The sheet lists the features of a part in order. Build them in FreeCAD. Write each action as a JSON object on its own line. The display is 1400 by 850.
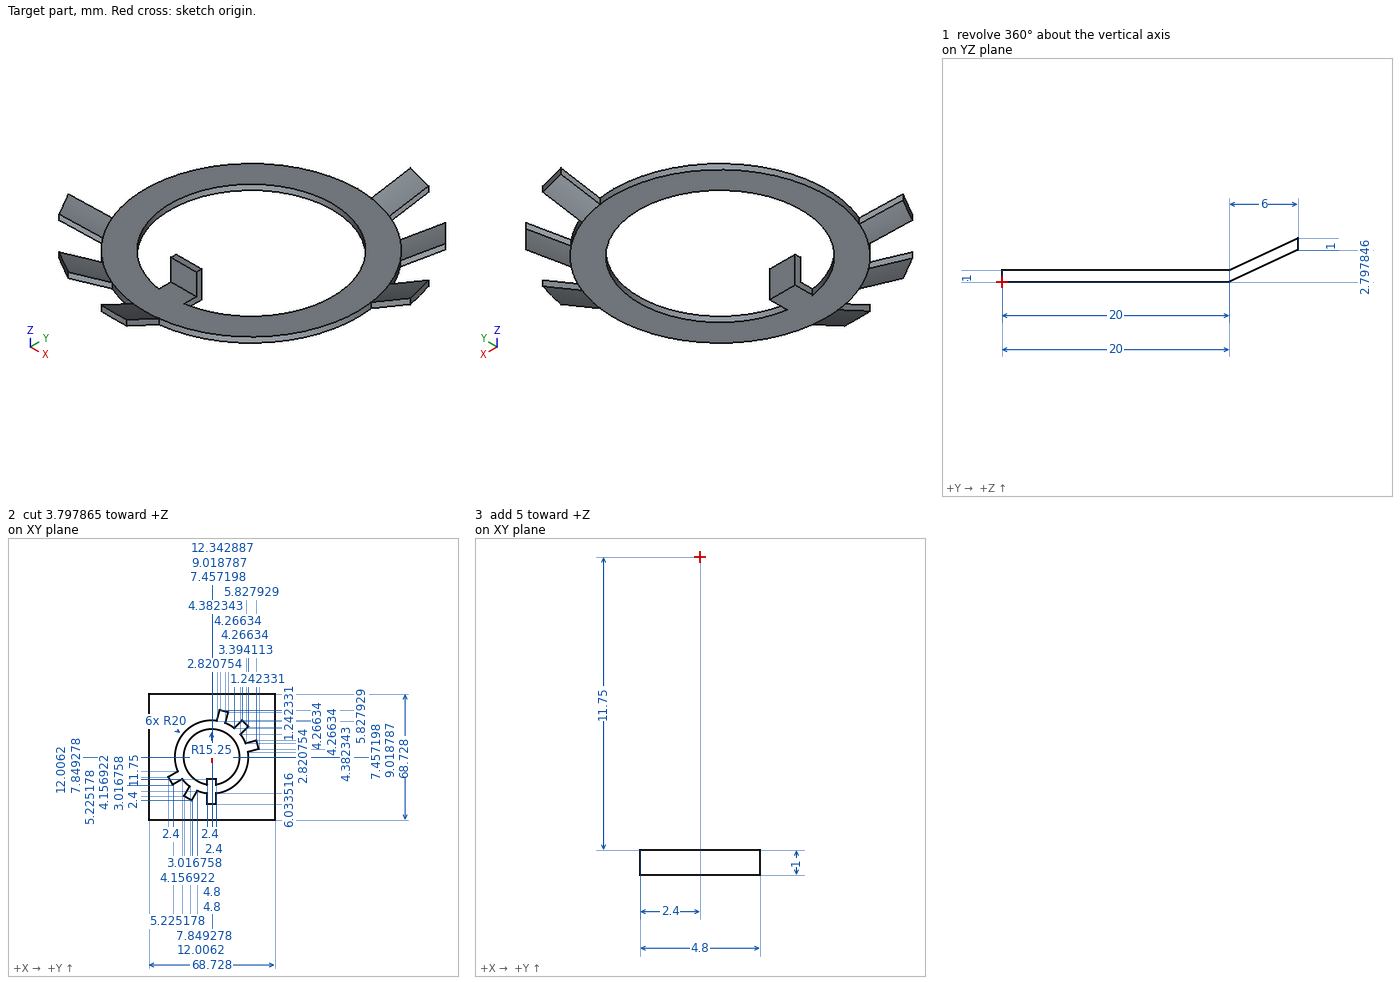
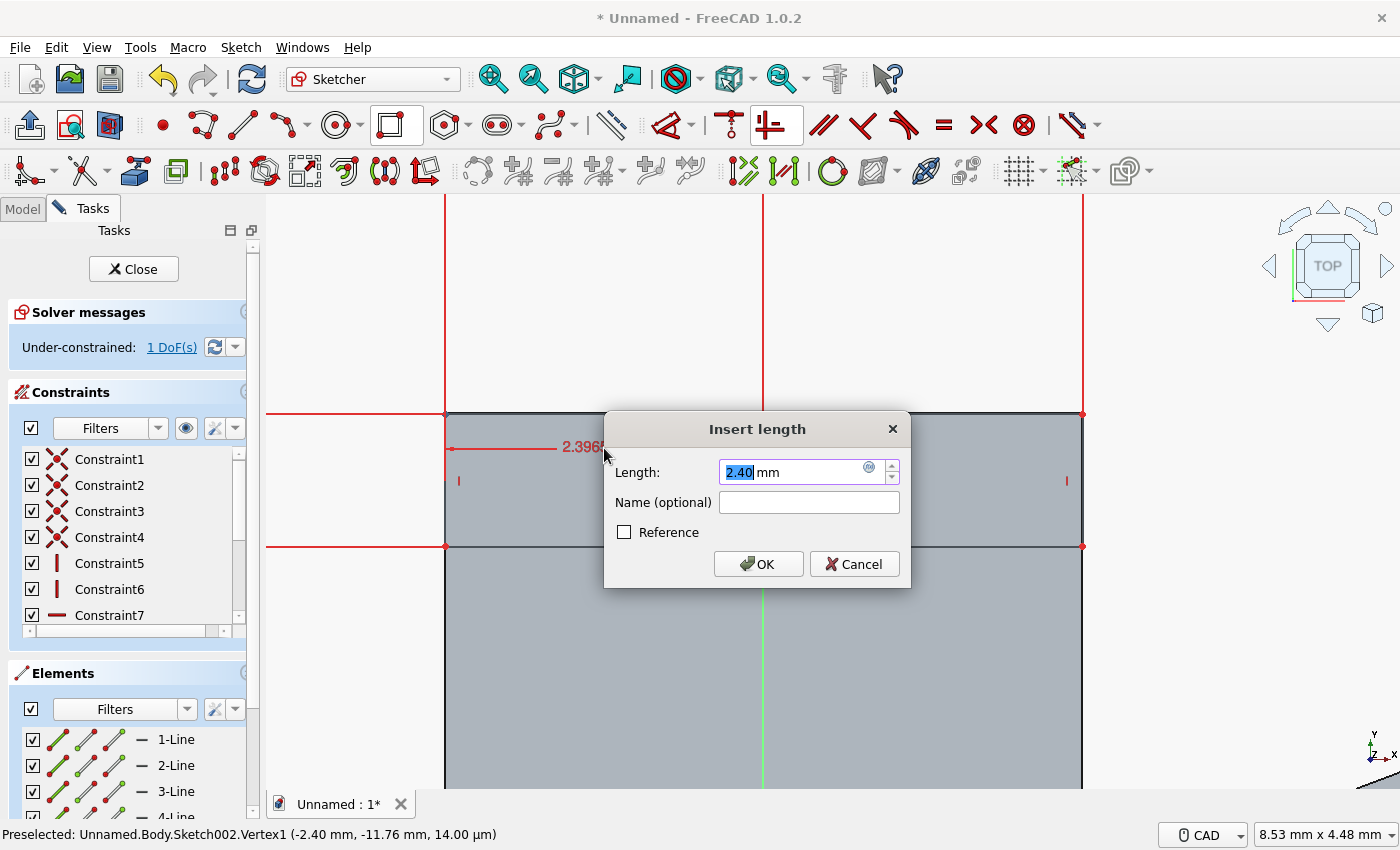
{"action": "type", "text": "2.4"}
{"action": "key", "text": "Return"}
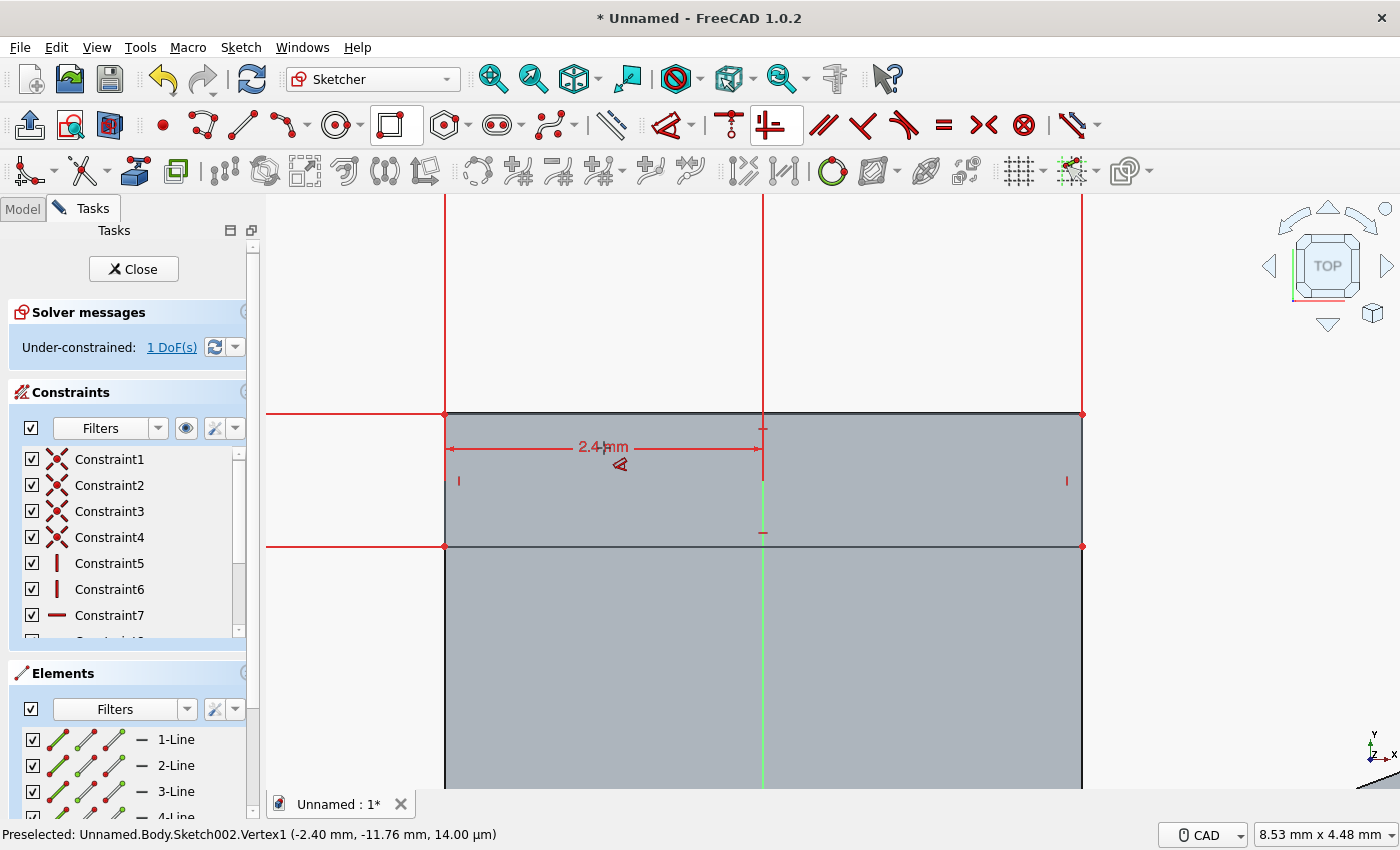
{"action": "left_click", "coordinate": [445, 414]}
{"action": "left_click", "coordinate": [411, 318]}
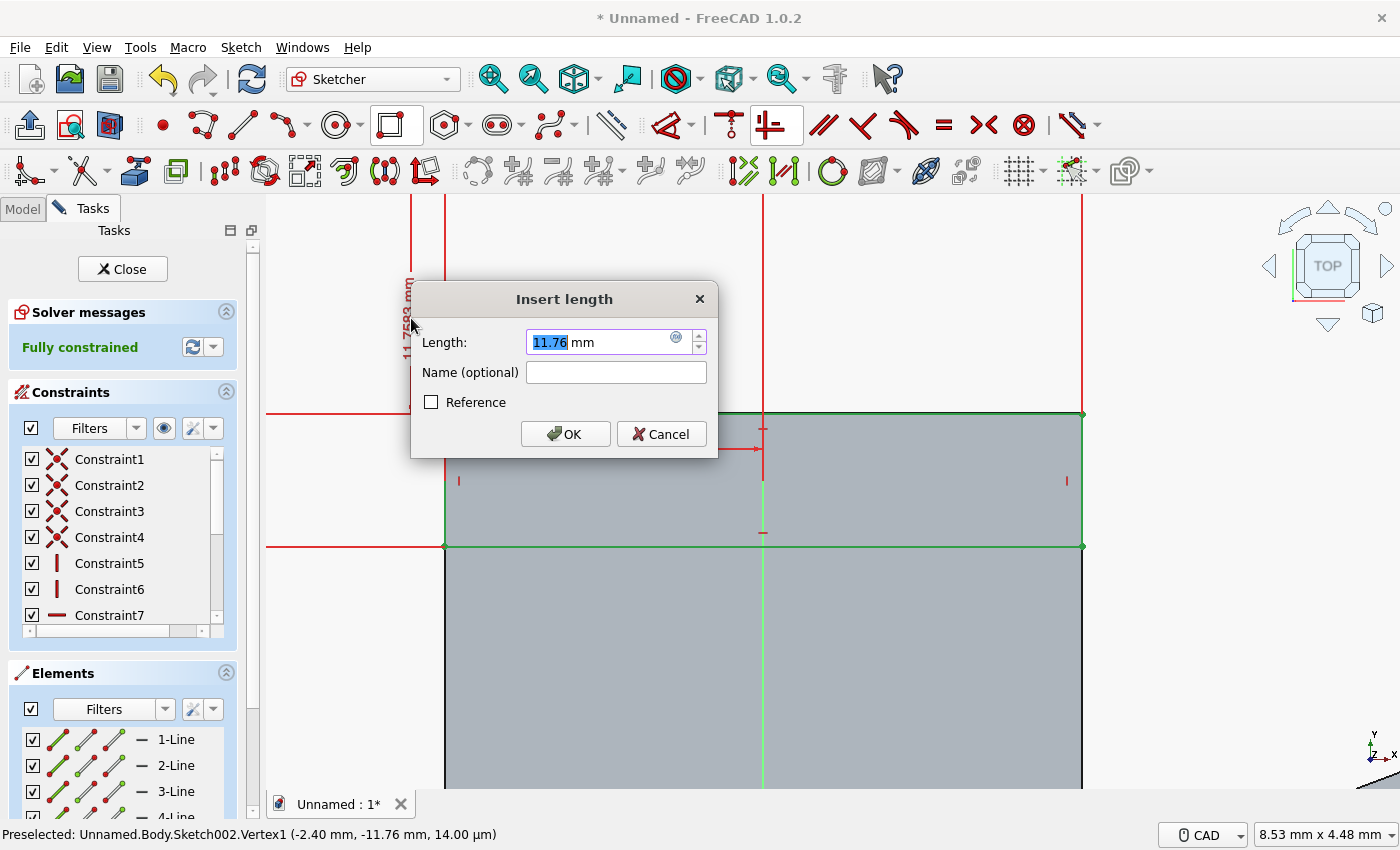
{"action": "type", "text": "11.75"}
{"action": "key", "text": "Return"}
{"action": "key", "text": "Escape"}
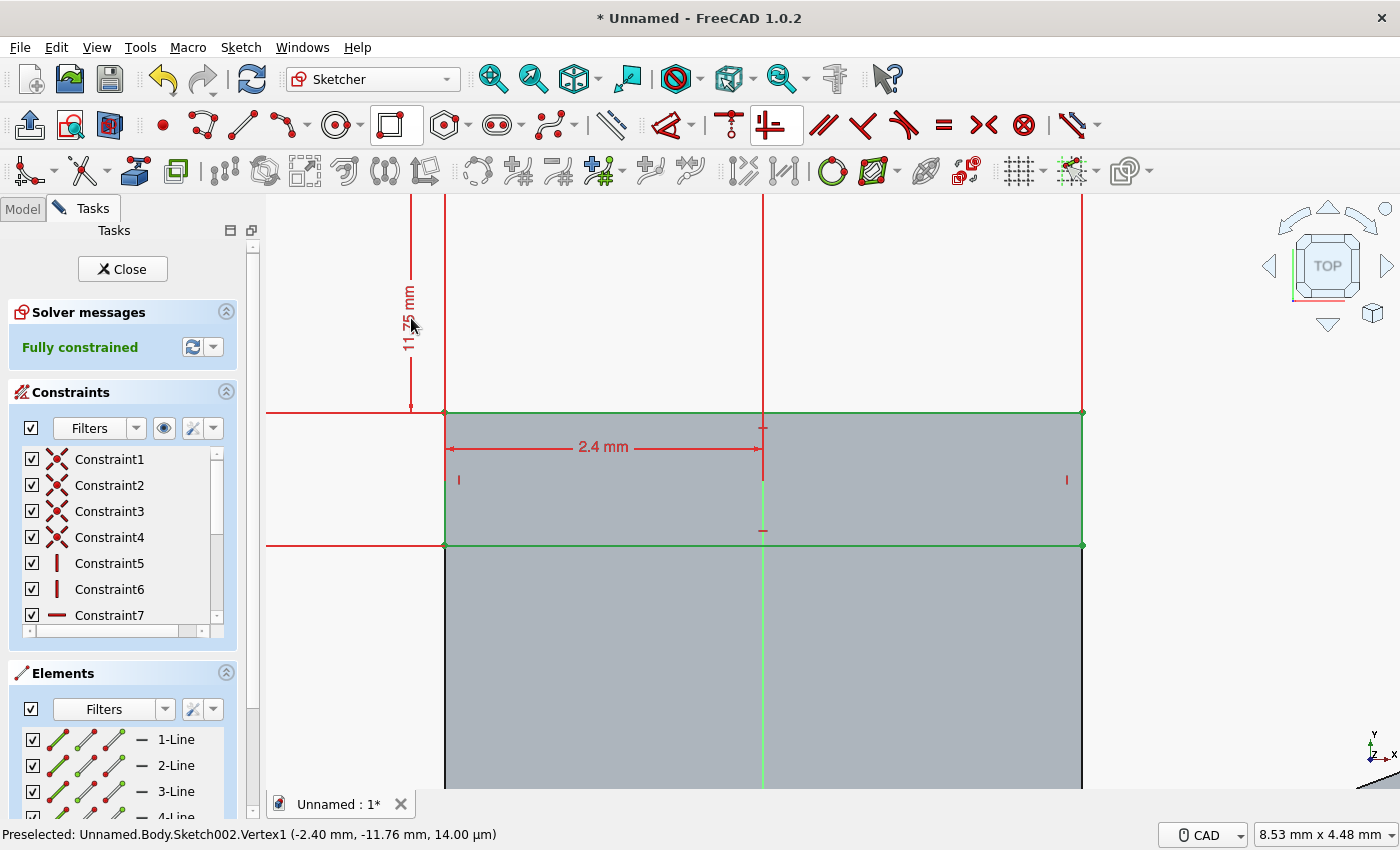
{"action": "left_click", "coordinate": [123, 269]}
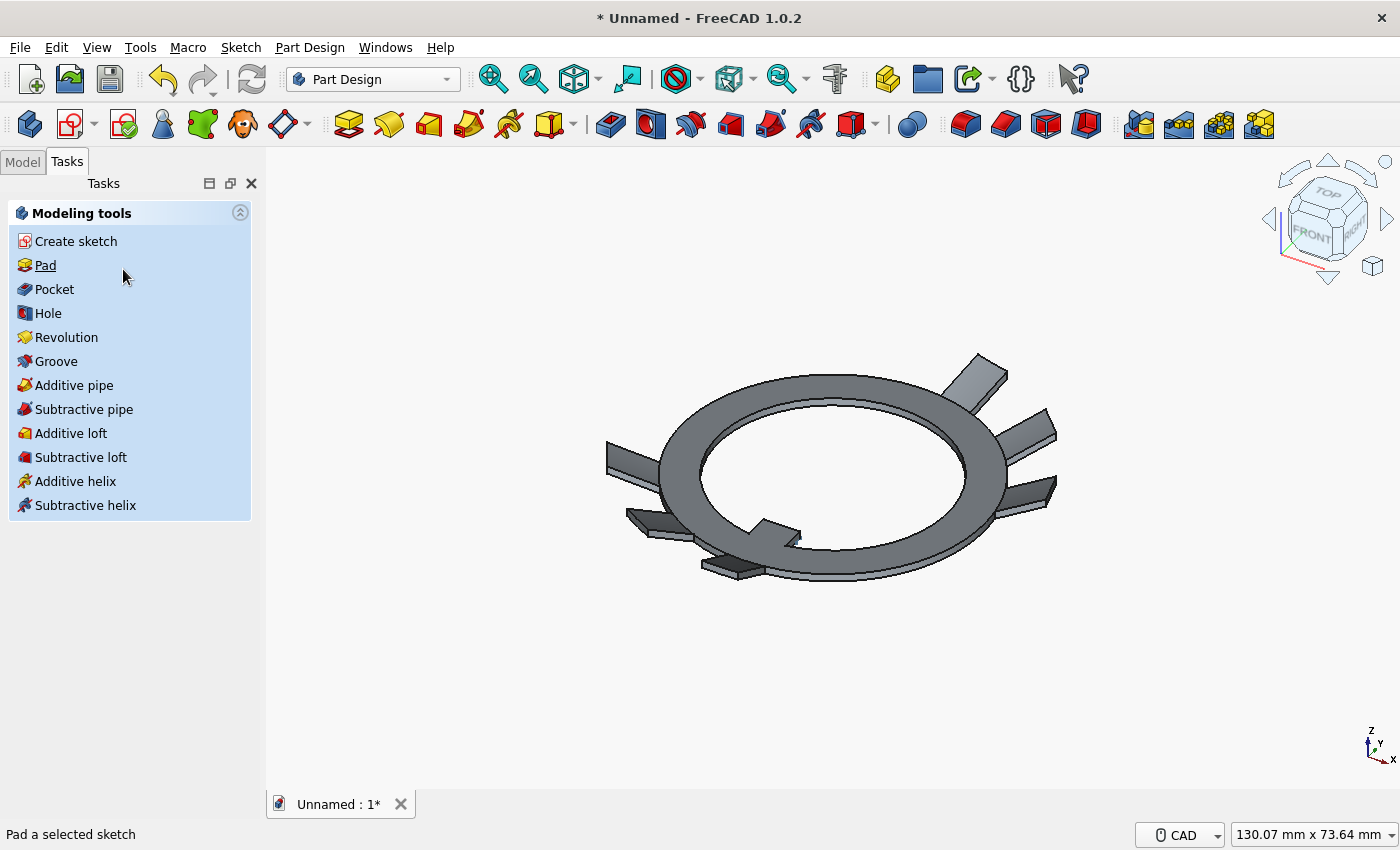
{"action": "left_click", "coordinate": [350, 124]}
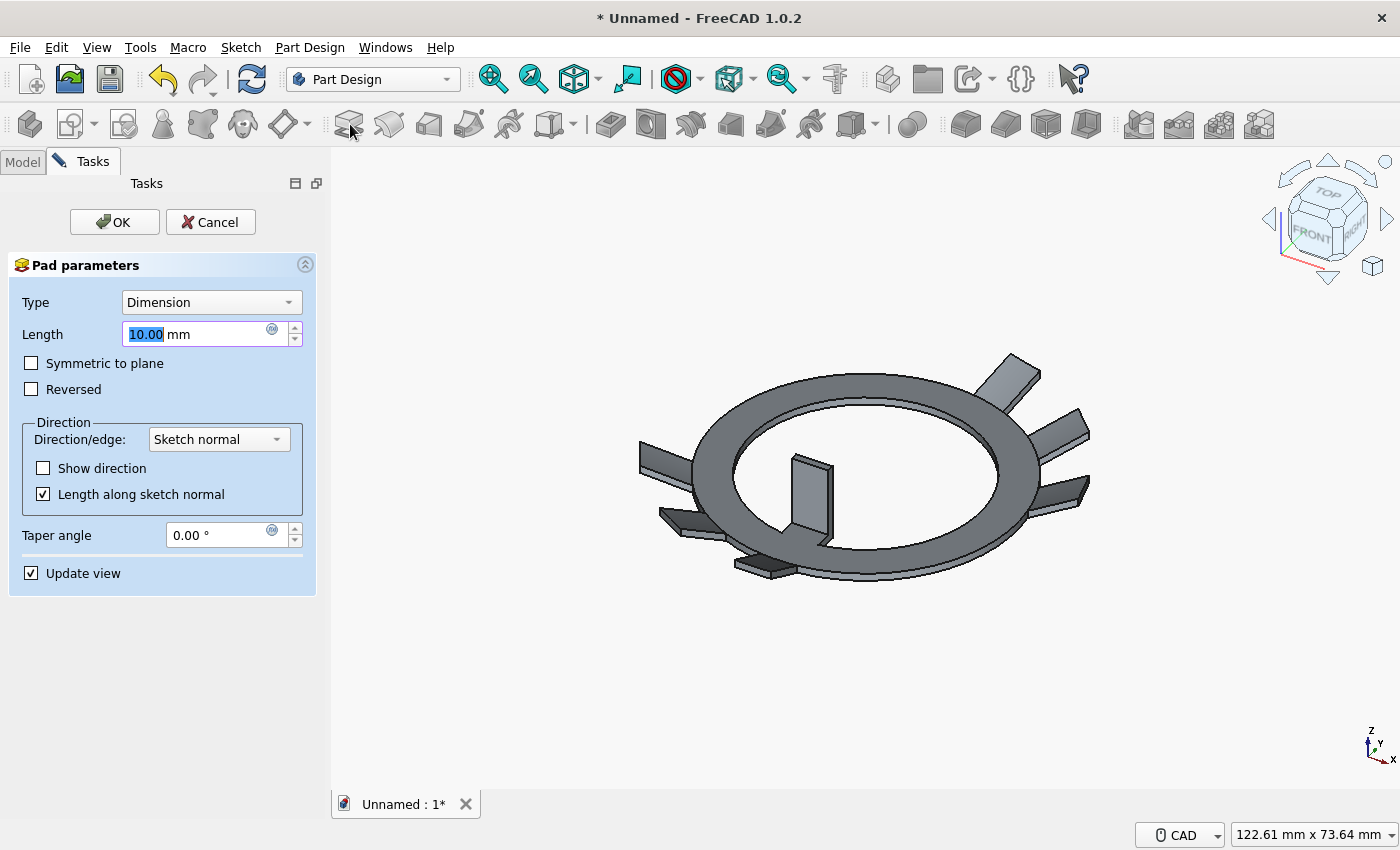
{"action": "type", "text": "5"}
{"action": "key", "text": "Tab"}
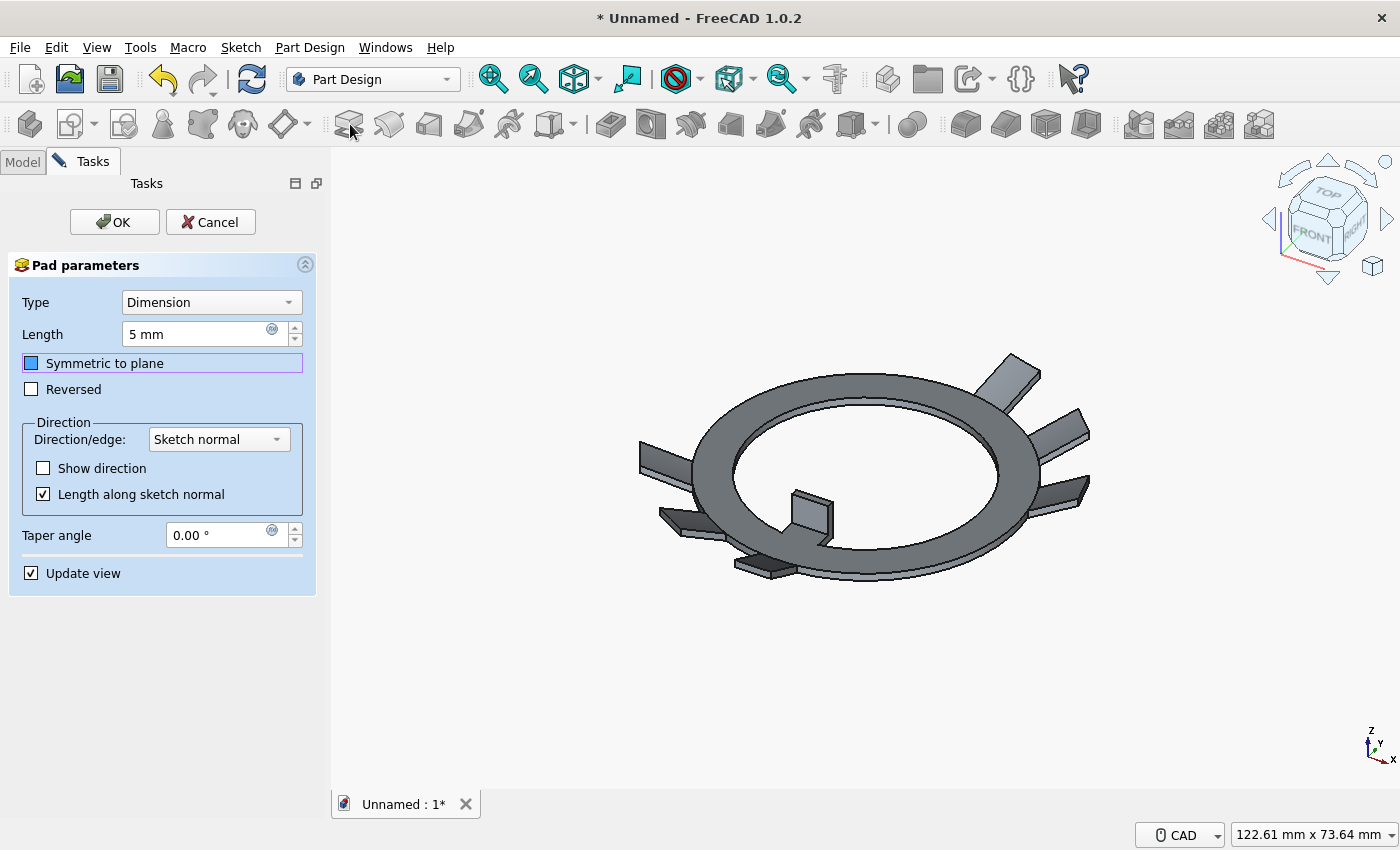
{"action": "left_click", "coordinate": [115, 222]}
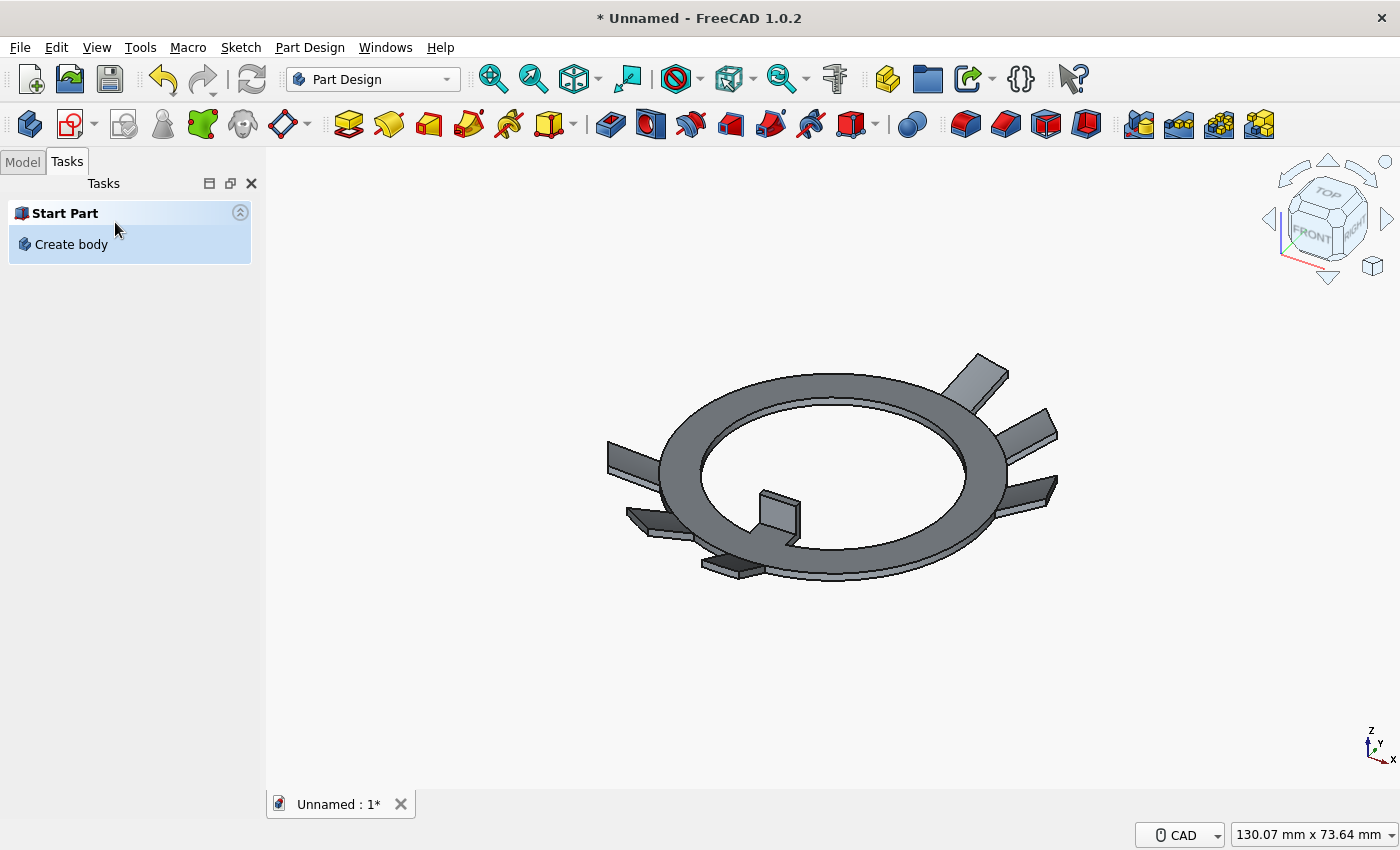
{"action": "key", "text": "0"}